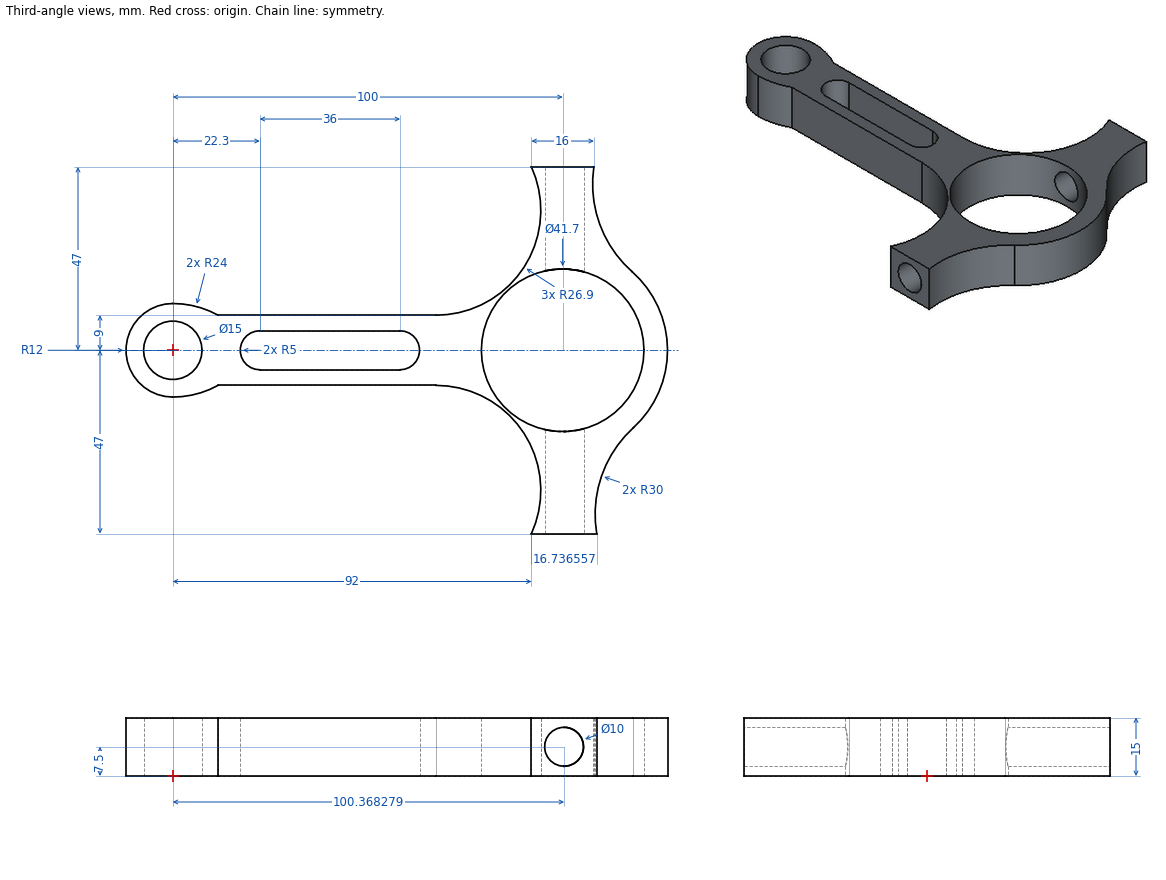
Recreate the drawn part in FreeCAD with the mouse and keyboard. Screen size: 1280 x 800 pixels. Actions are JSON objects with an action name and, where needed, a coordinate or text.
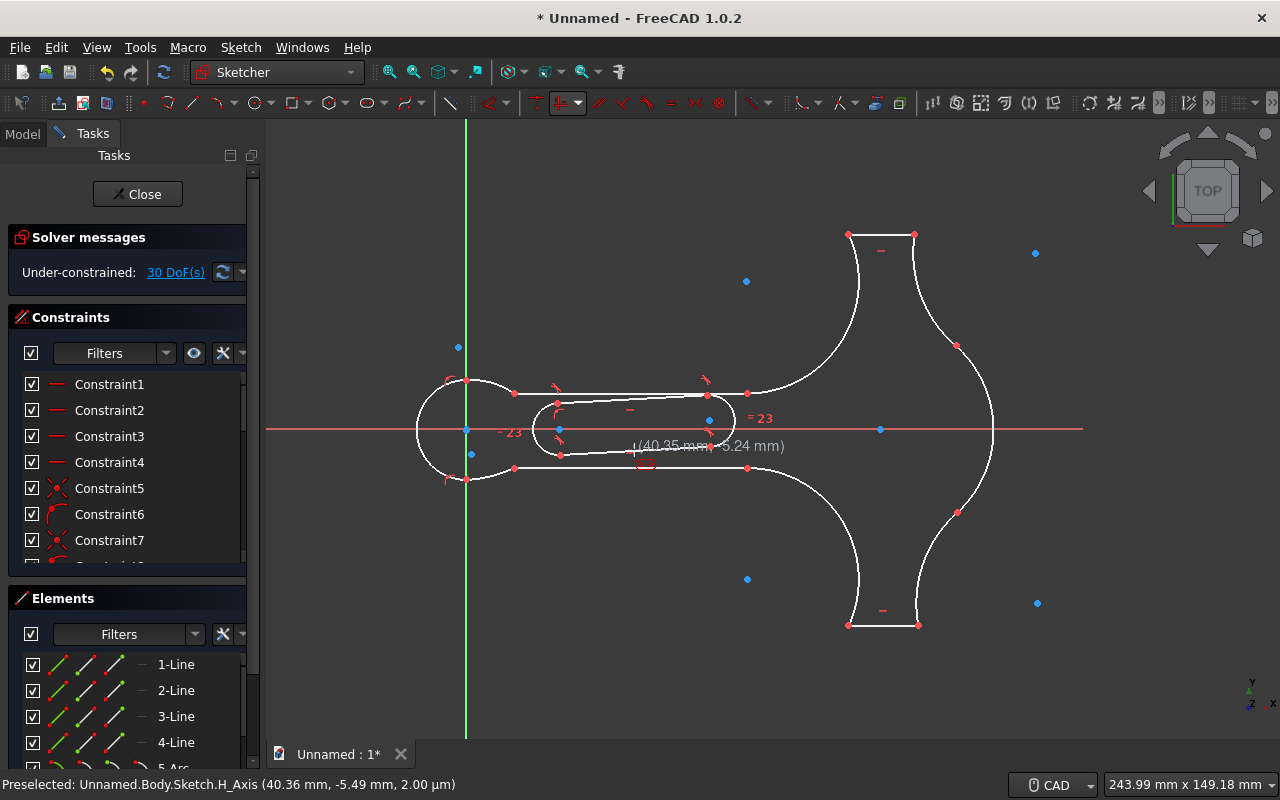
{"action": "left_click", "coordinate": [256, 104]}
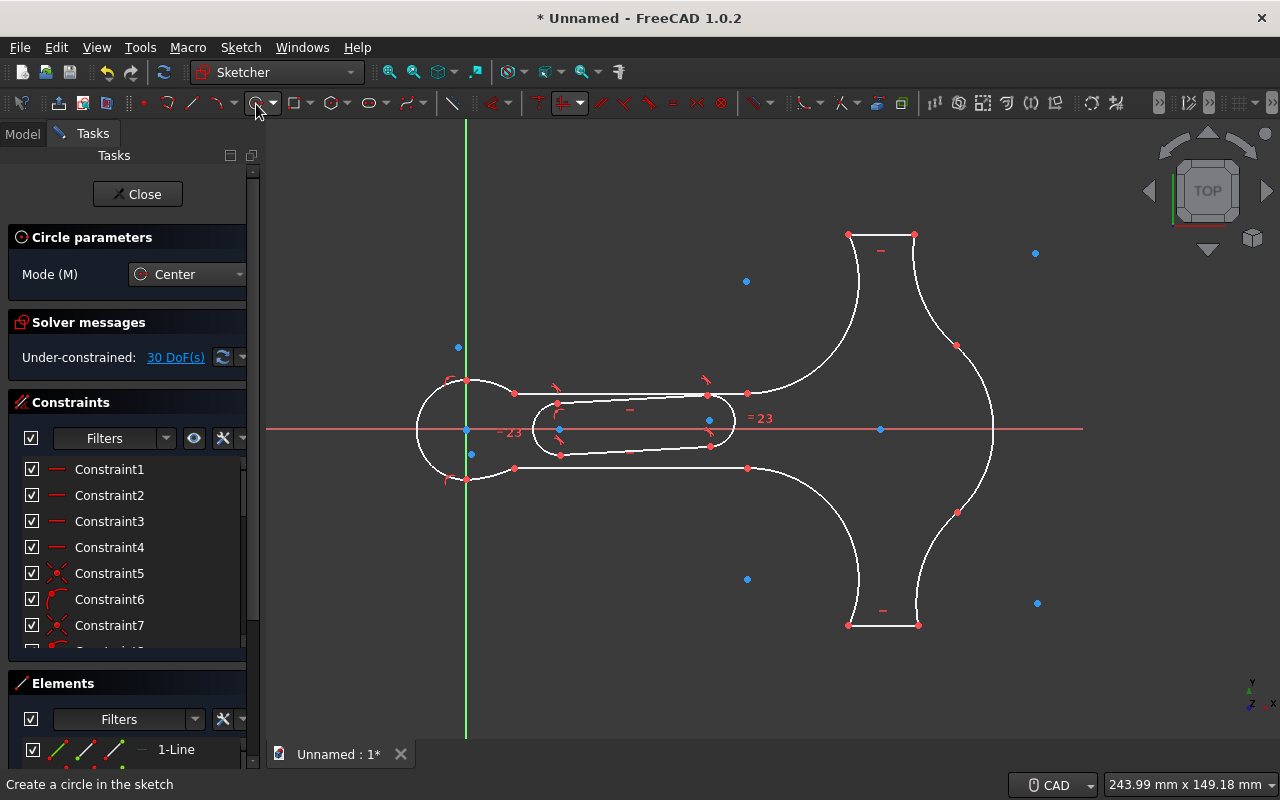
{"action": "left_click", "coordinate": [466, 429]}
{"action": "left_click", "coordinate": [488, 407]}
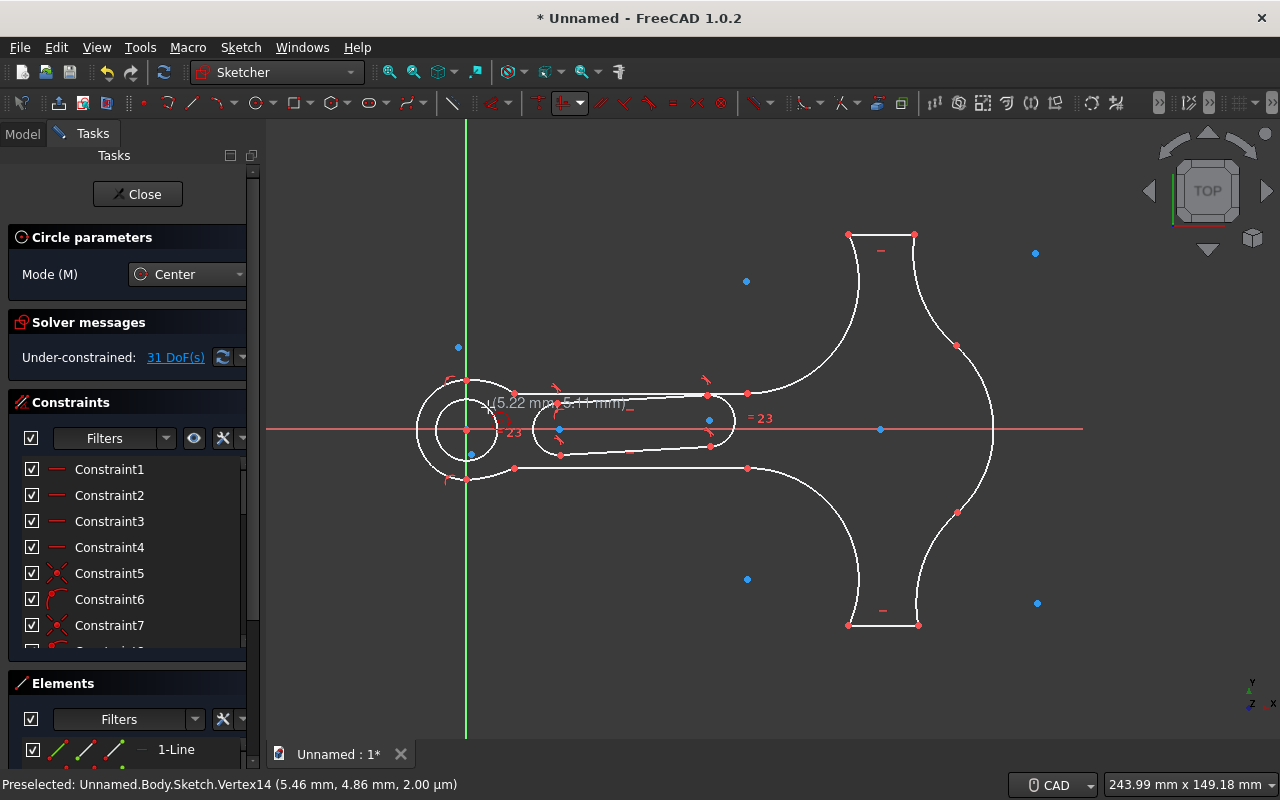
{"action": "left_click", "coordinate": [882, 429]}
{"action": "left_click", "coordinate": [943, 368]}
{"action": "key", "text": "Escape"}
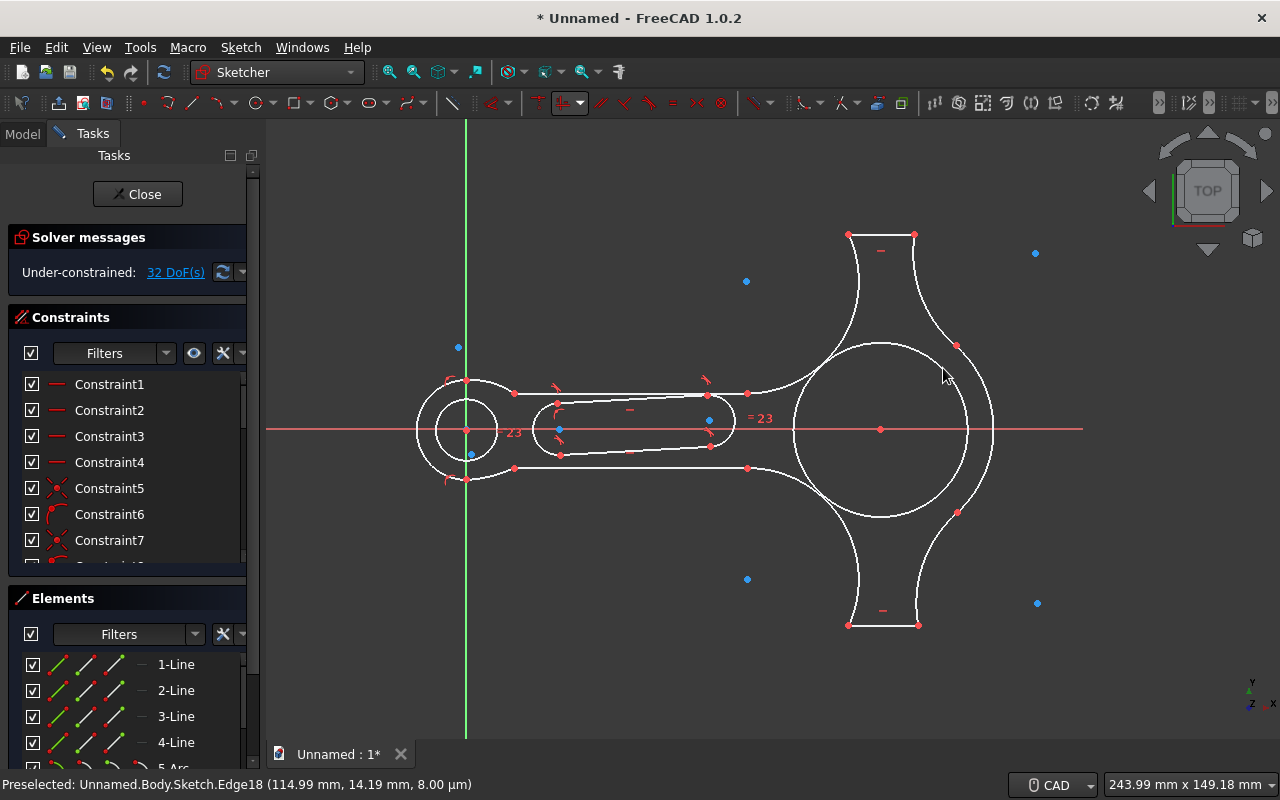
{"action": "scroll", "coordinate": [561, 394], "scroll_direction": "up", "scroll_amount": 2}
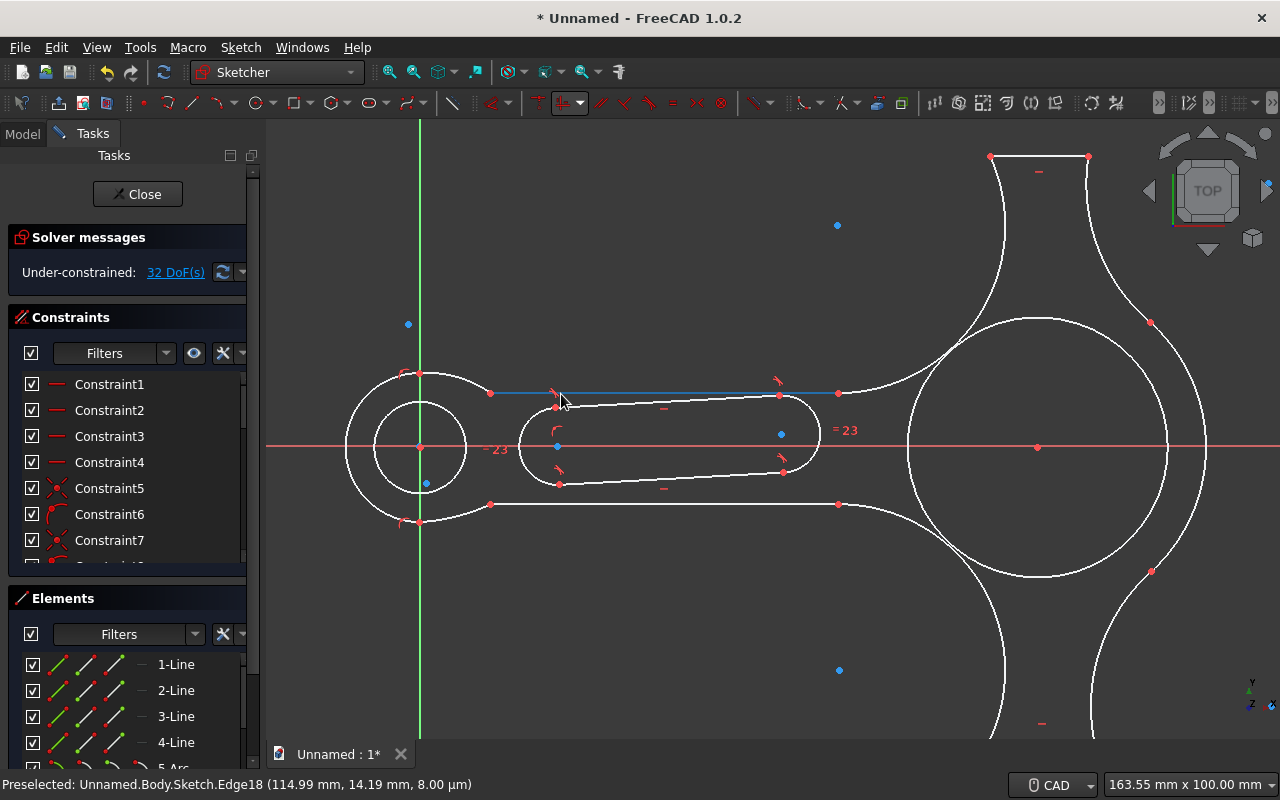
{"action": "left_click", "coordinate": [595, 393]}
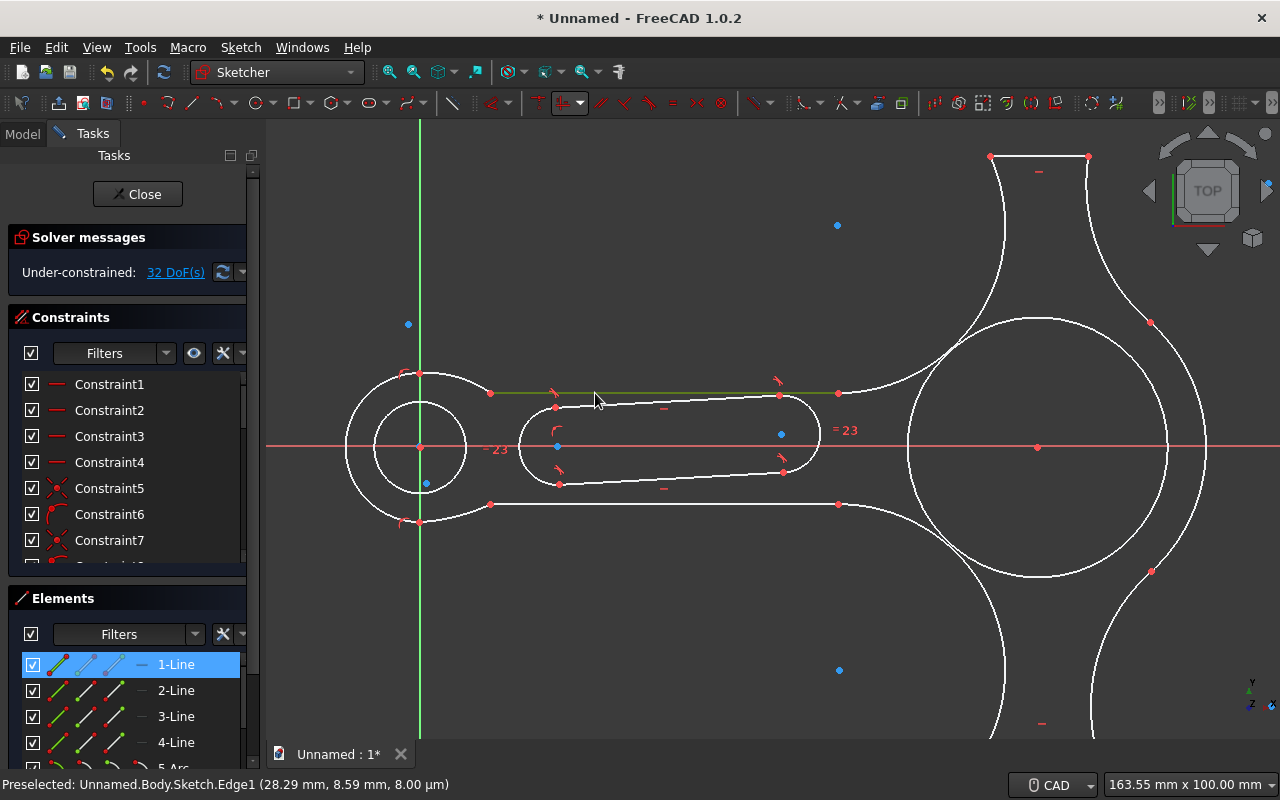
{"action": "left_click", "coordinate": [1003, 254]}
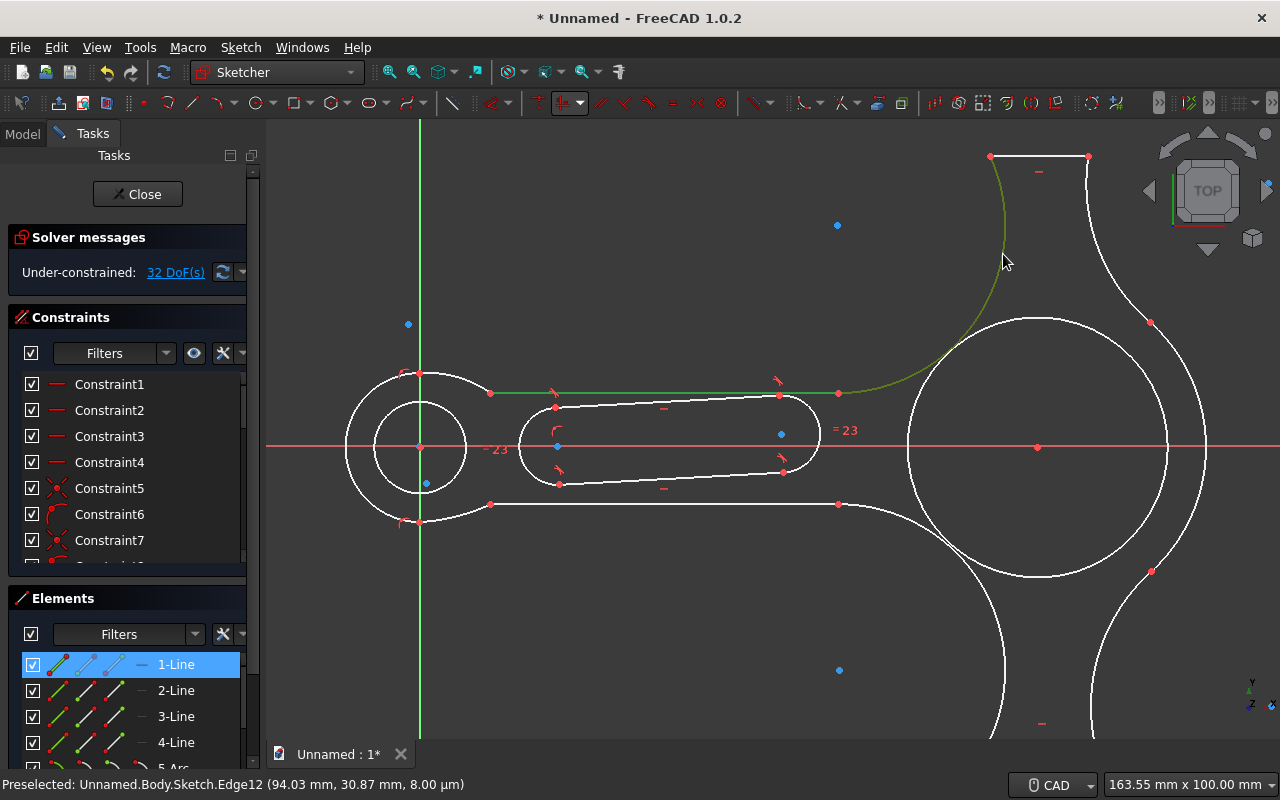
{"action": "left_click", "coordinate": [650, 104]}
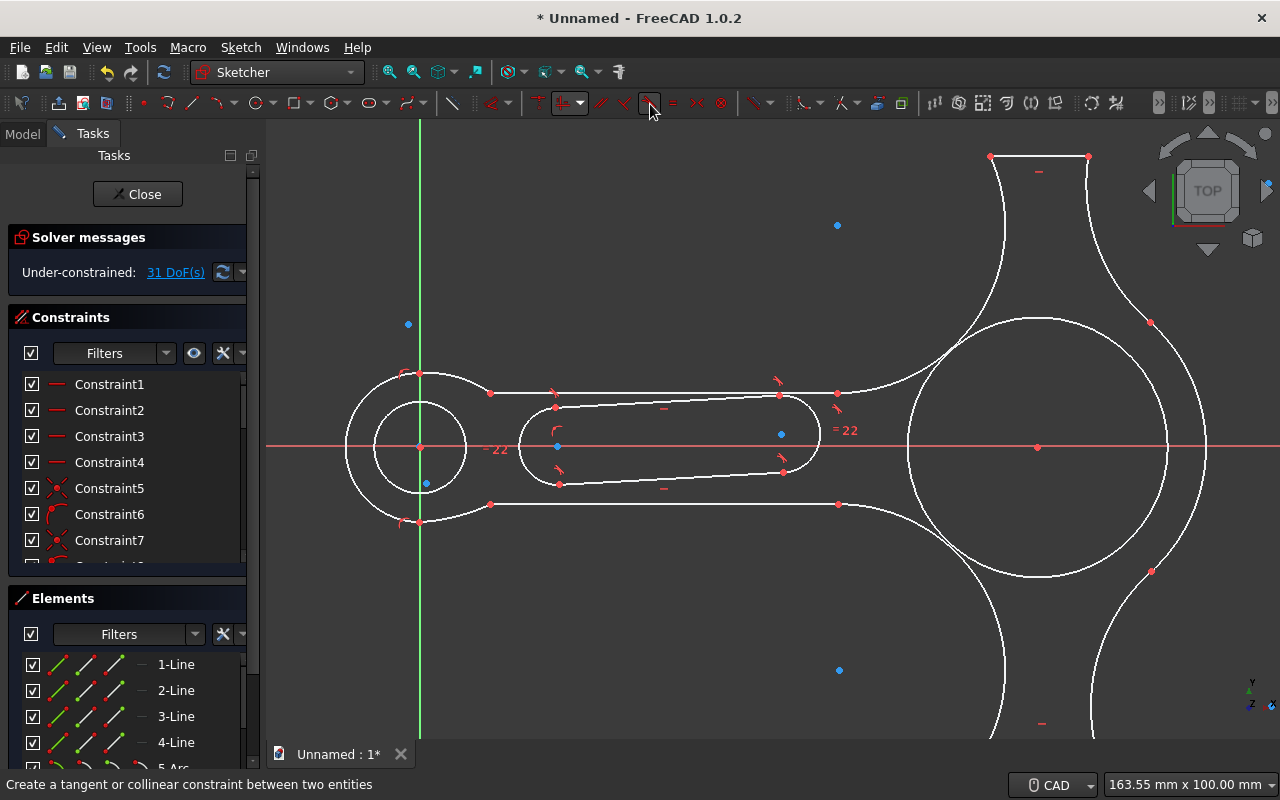
{"action": "left_click", "coordinate": [595, 504]}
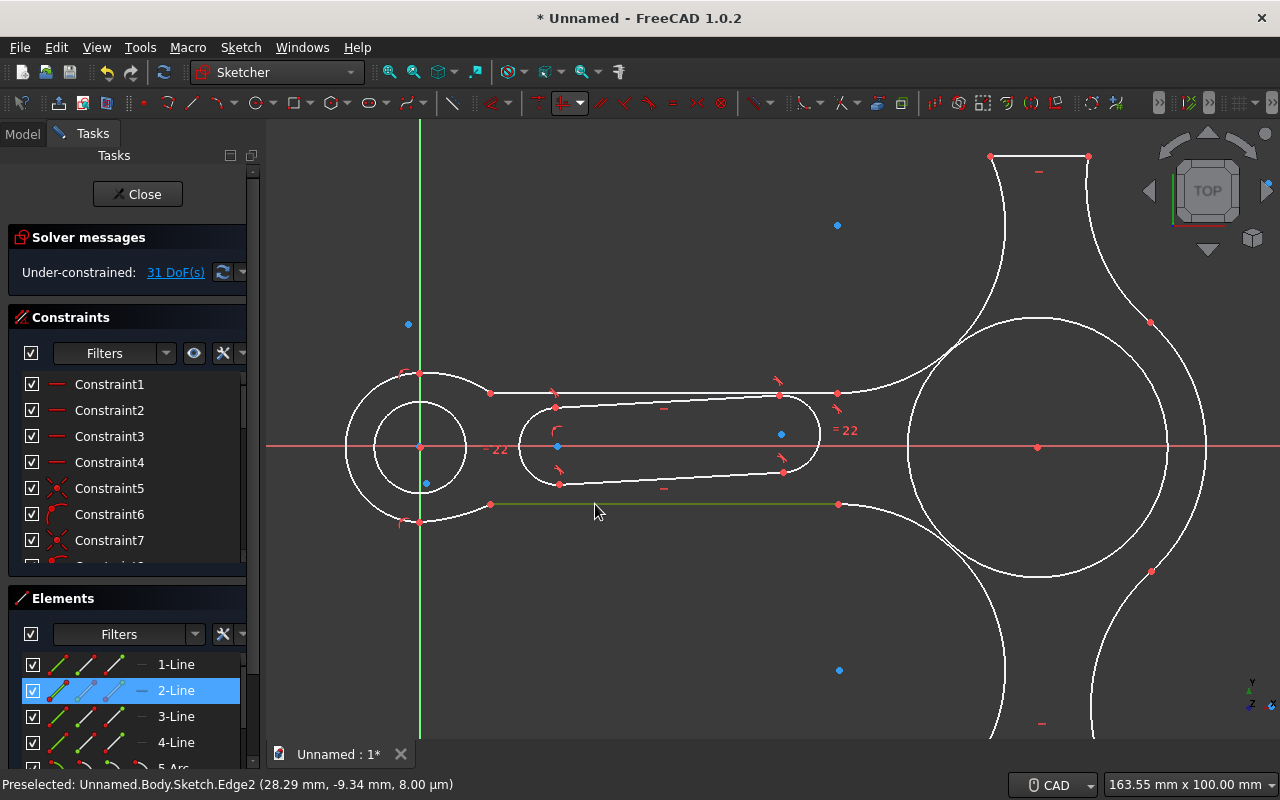
{"action": "left_click", "coordinate": [1003, 642]}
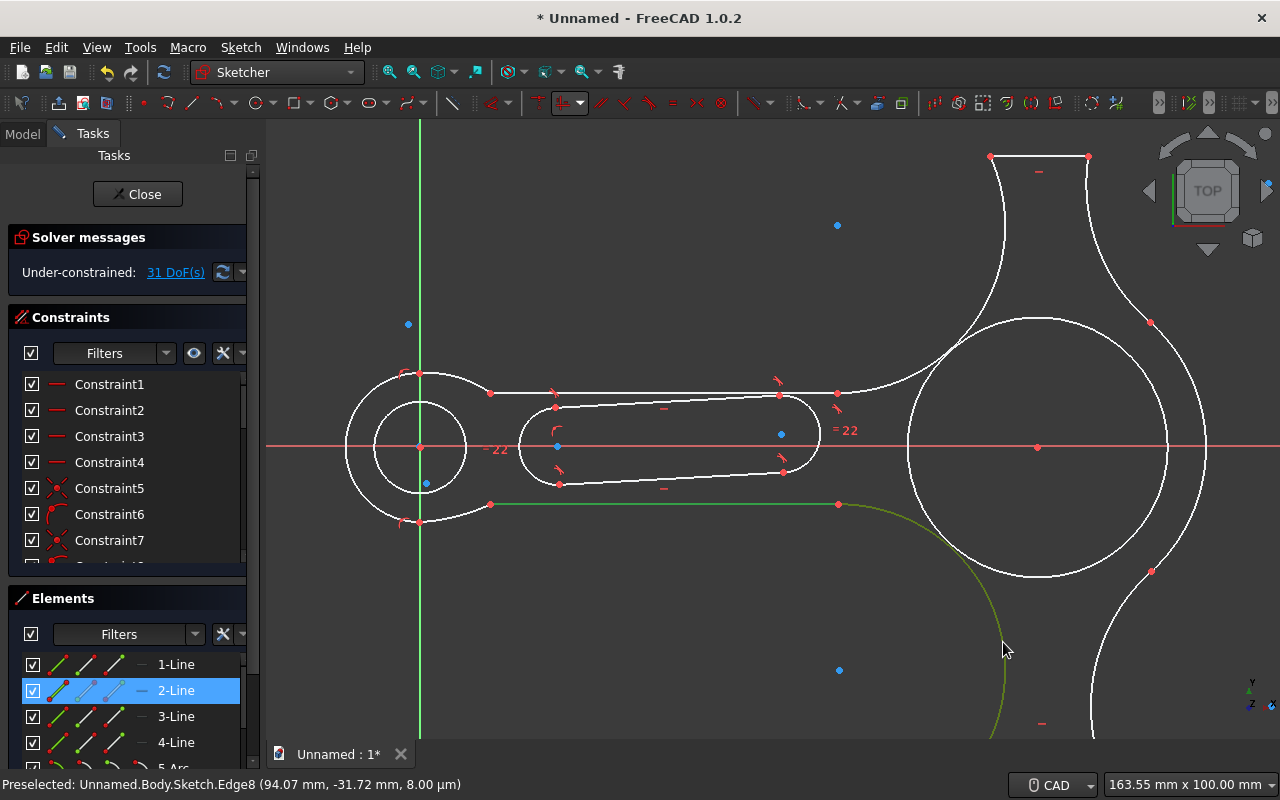
{"action": "left_click", "coordinate": [650, 104]}